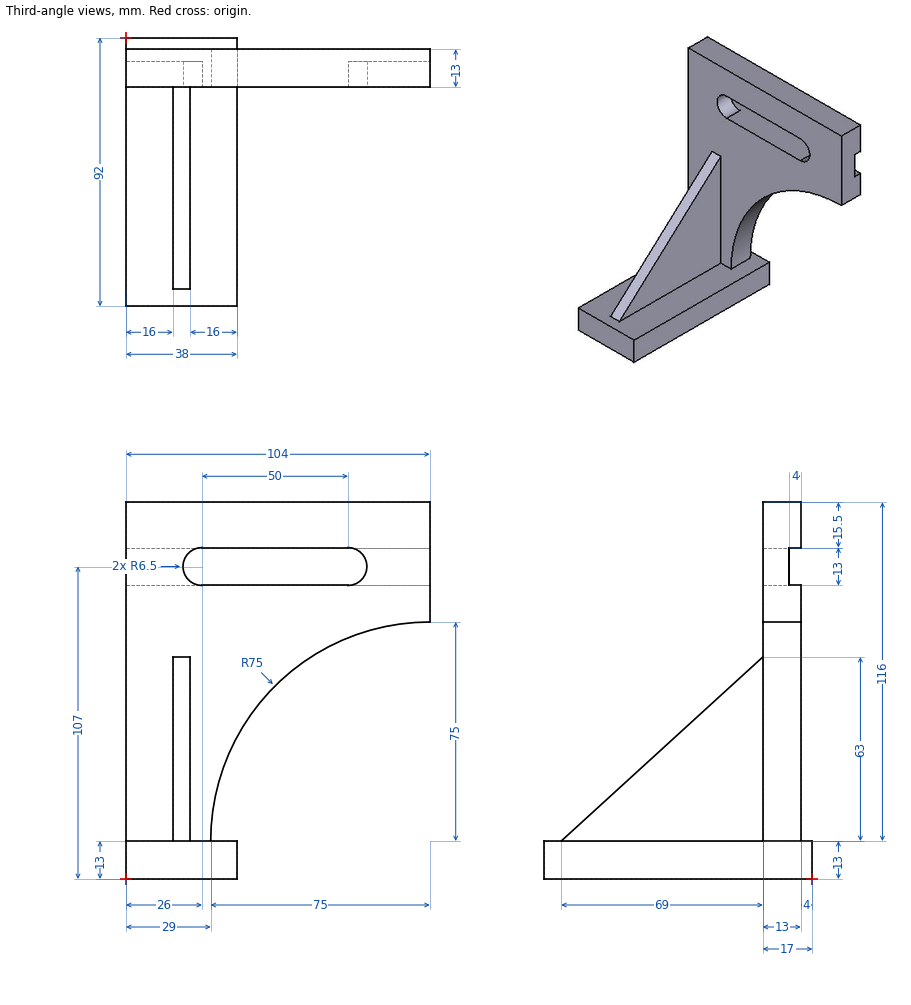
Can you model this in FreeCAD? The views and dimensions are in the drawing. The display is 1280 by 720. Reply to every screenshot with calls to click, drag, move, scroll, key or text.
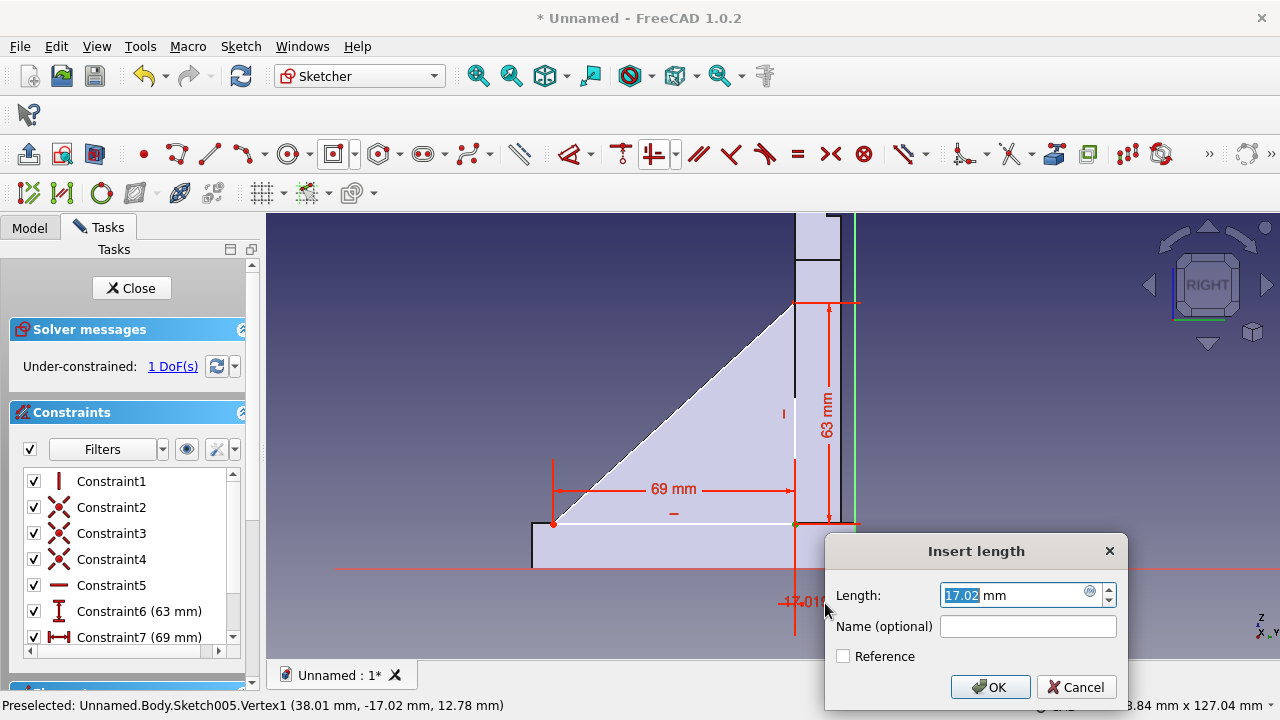
text(17)
key(Return)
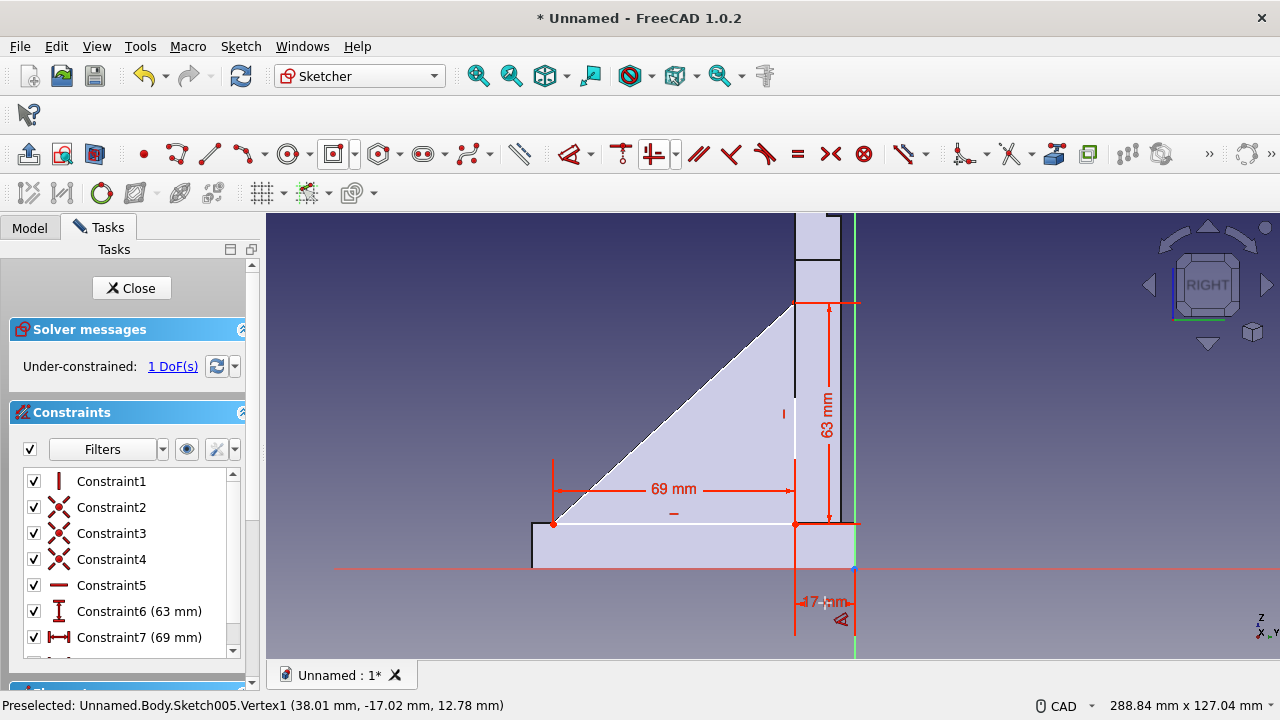
click(795, 524)
click(889, 547)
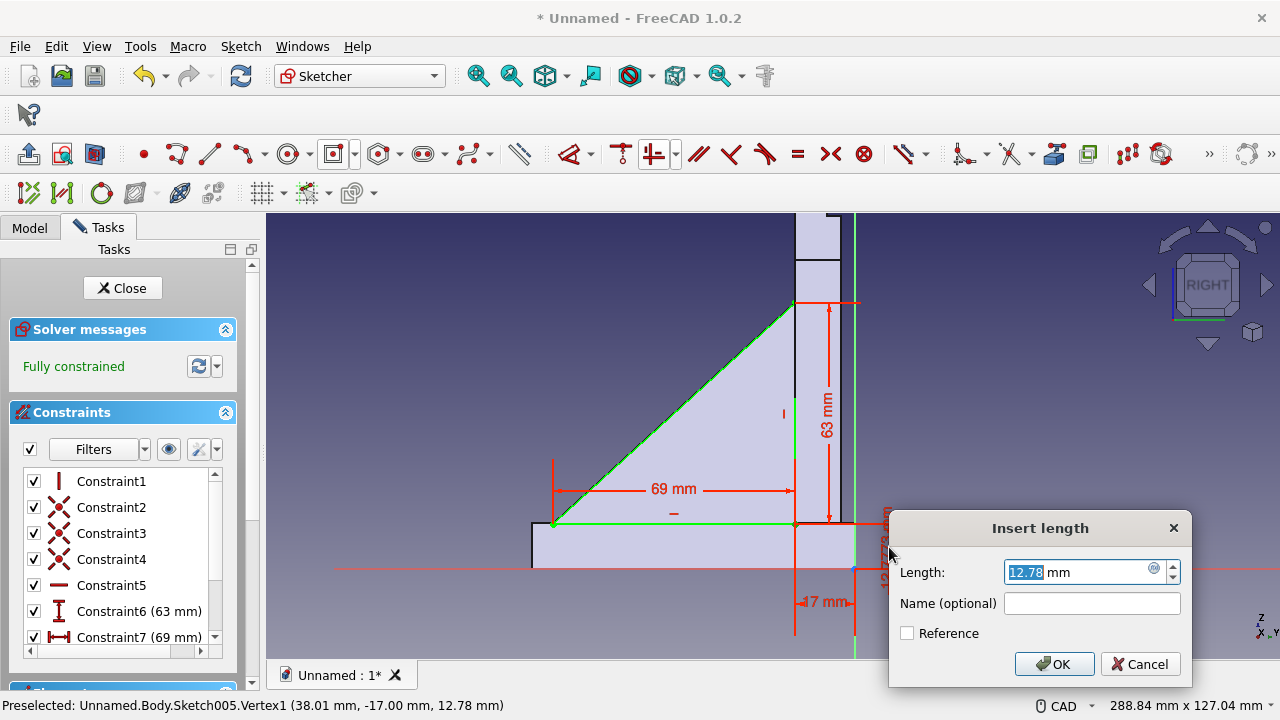
text(13)
key(Return)
key(Escape)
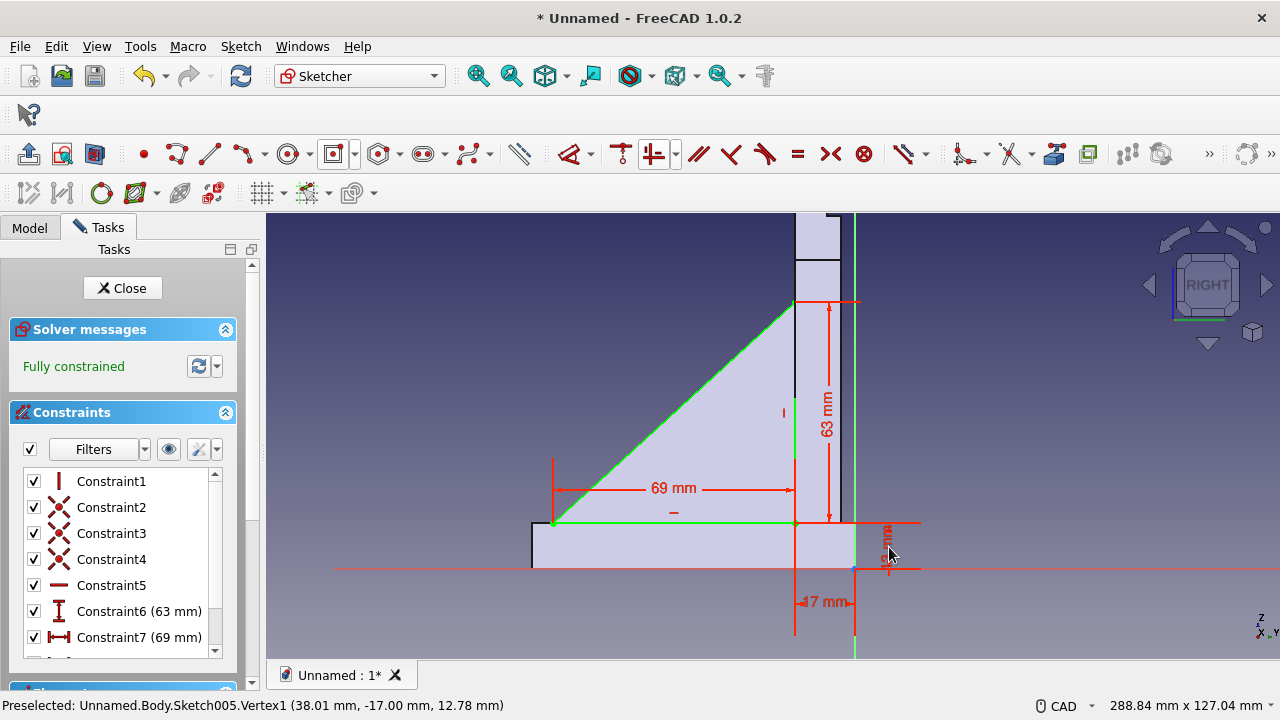
click(123, 288)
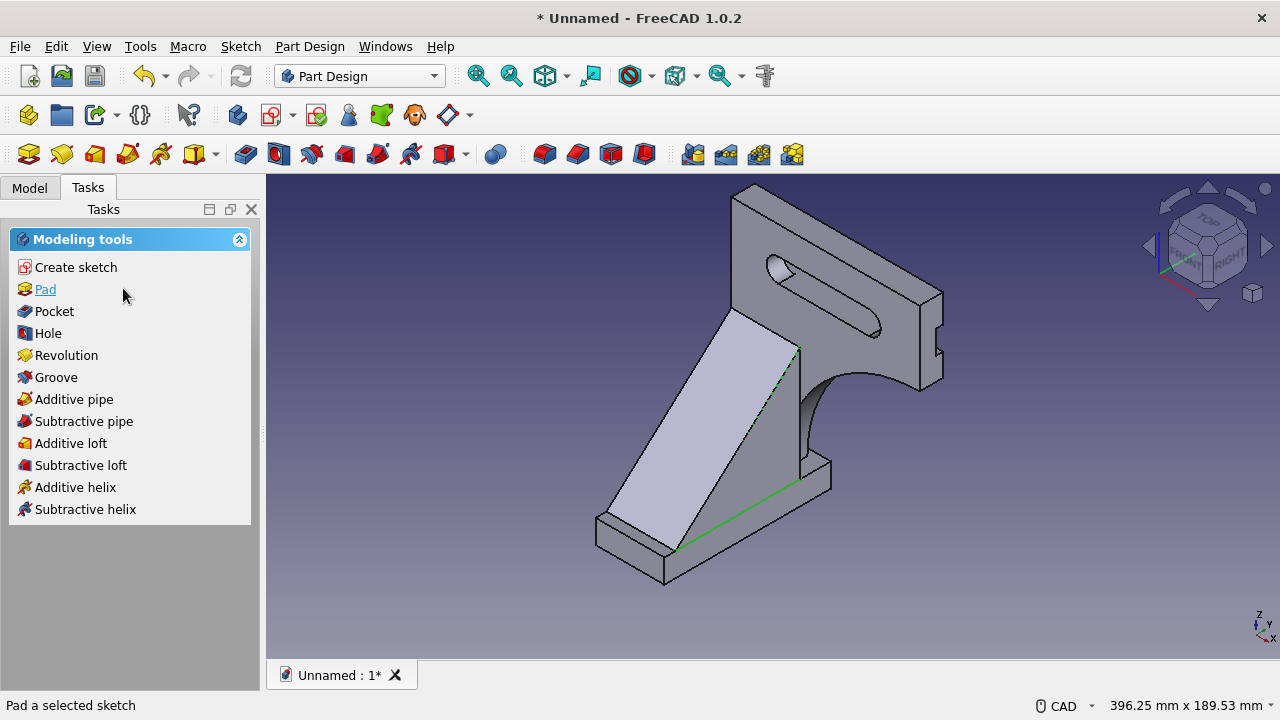
click(246, 154)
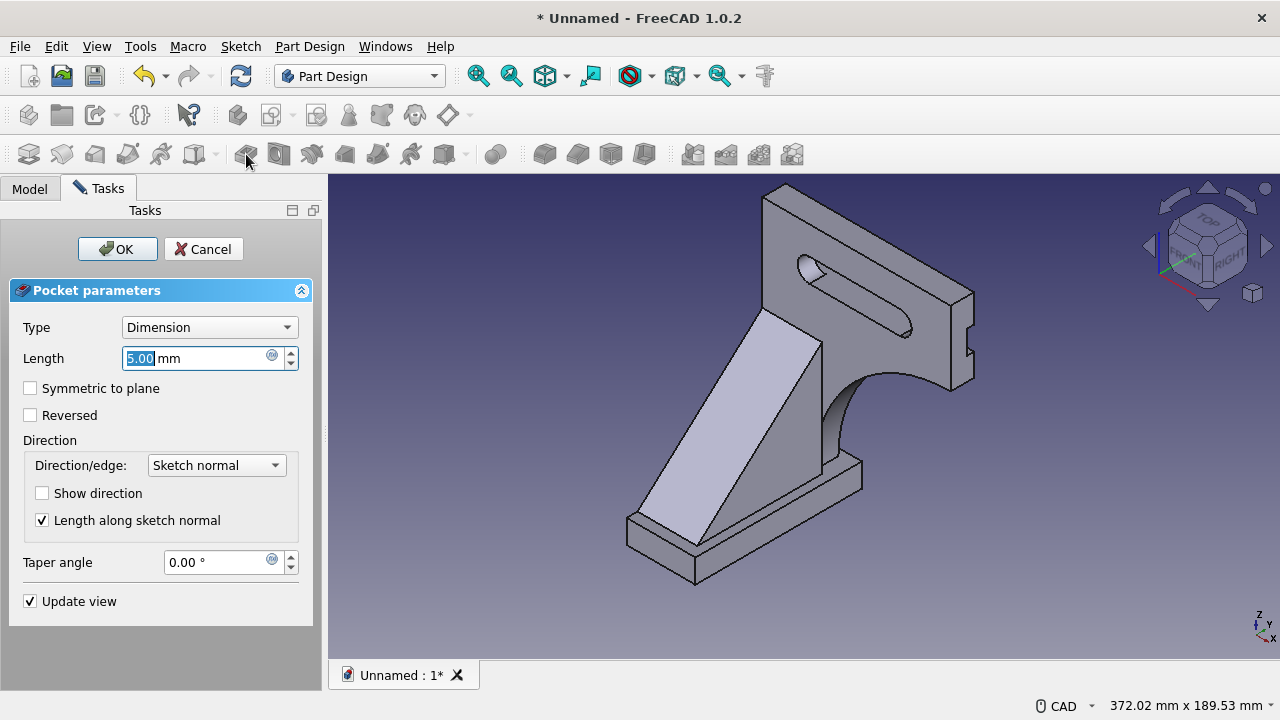
text(16)
key(Tab)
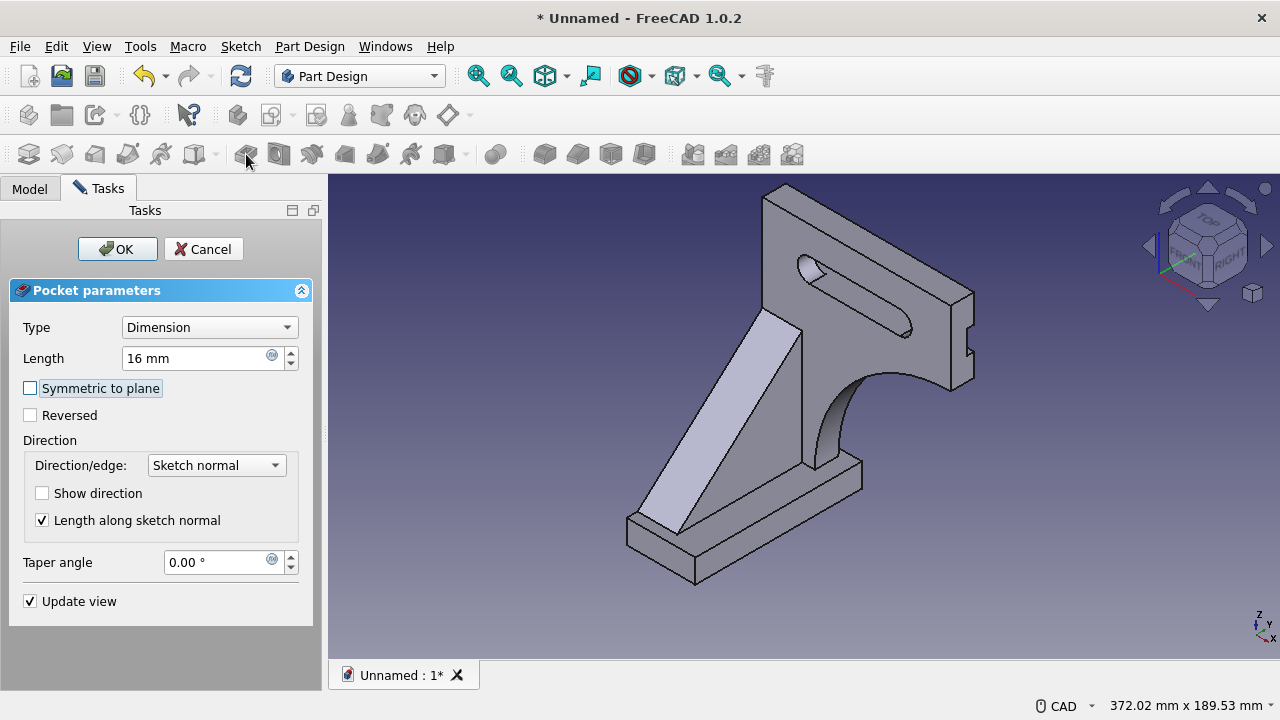
click(118, 249)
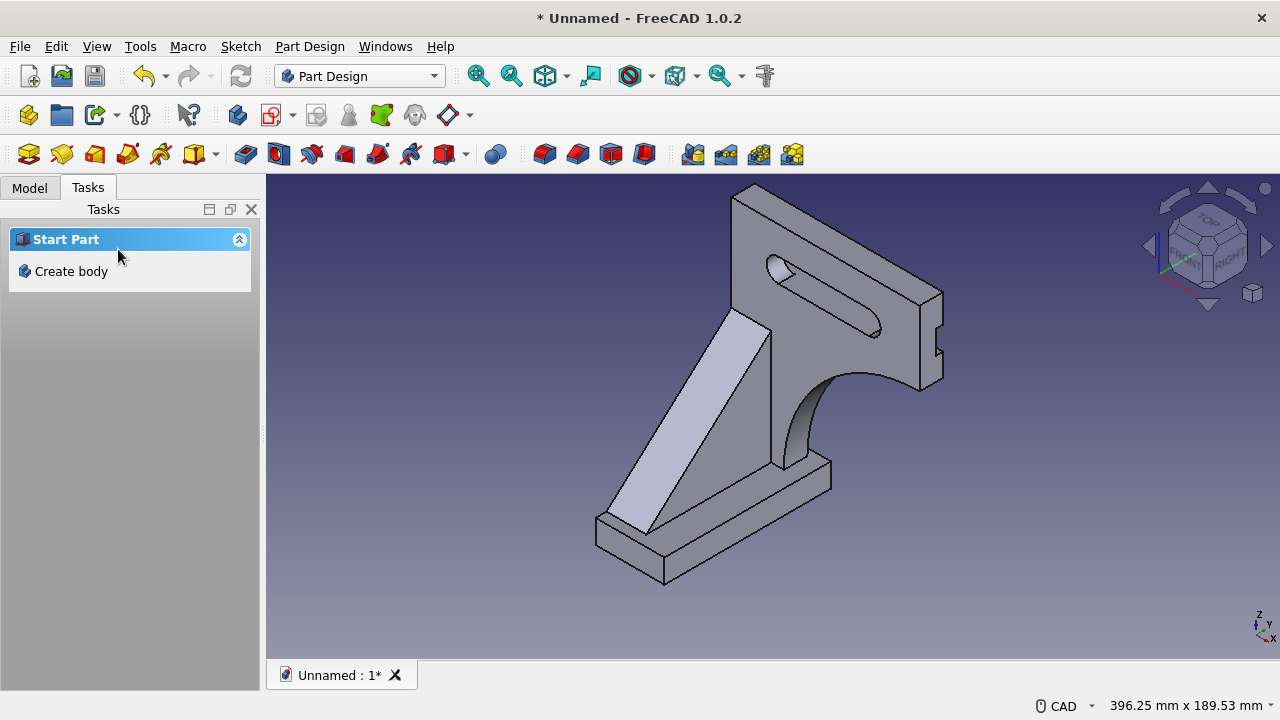
key(6)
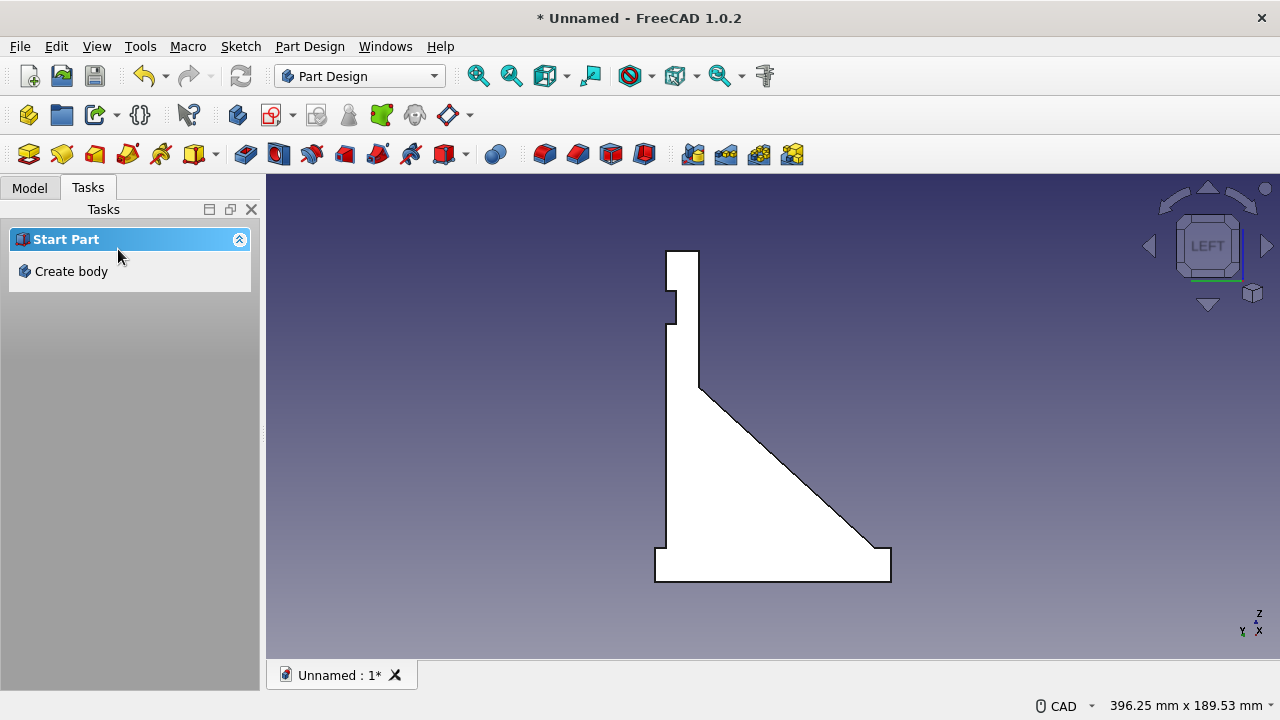
click(739, 510)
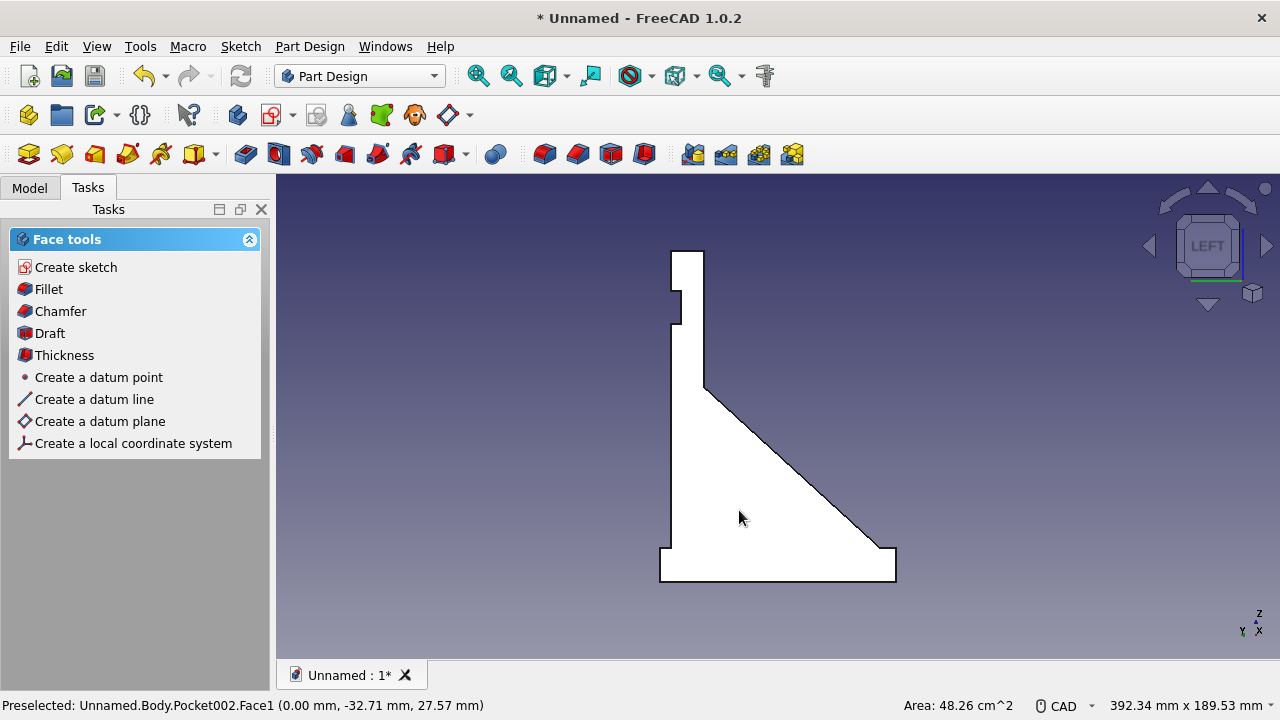
click(270, 116)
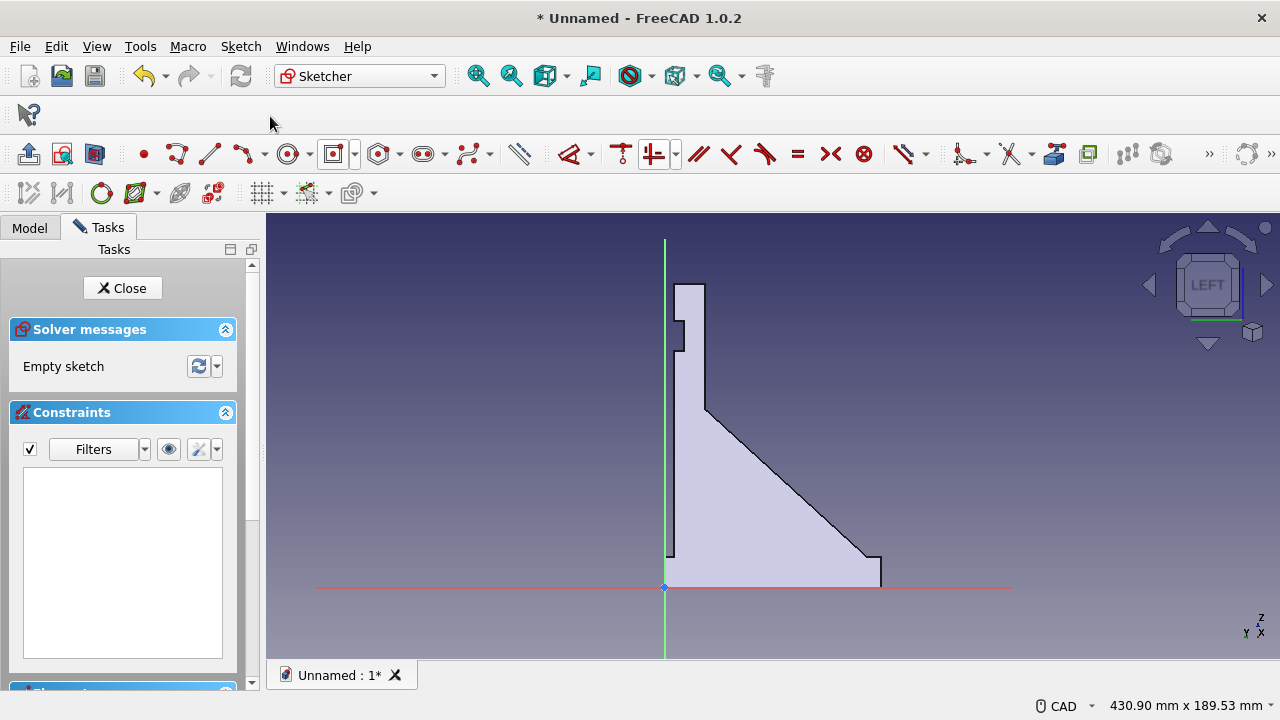
scroll(891, 625, up, 2)